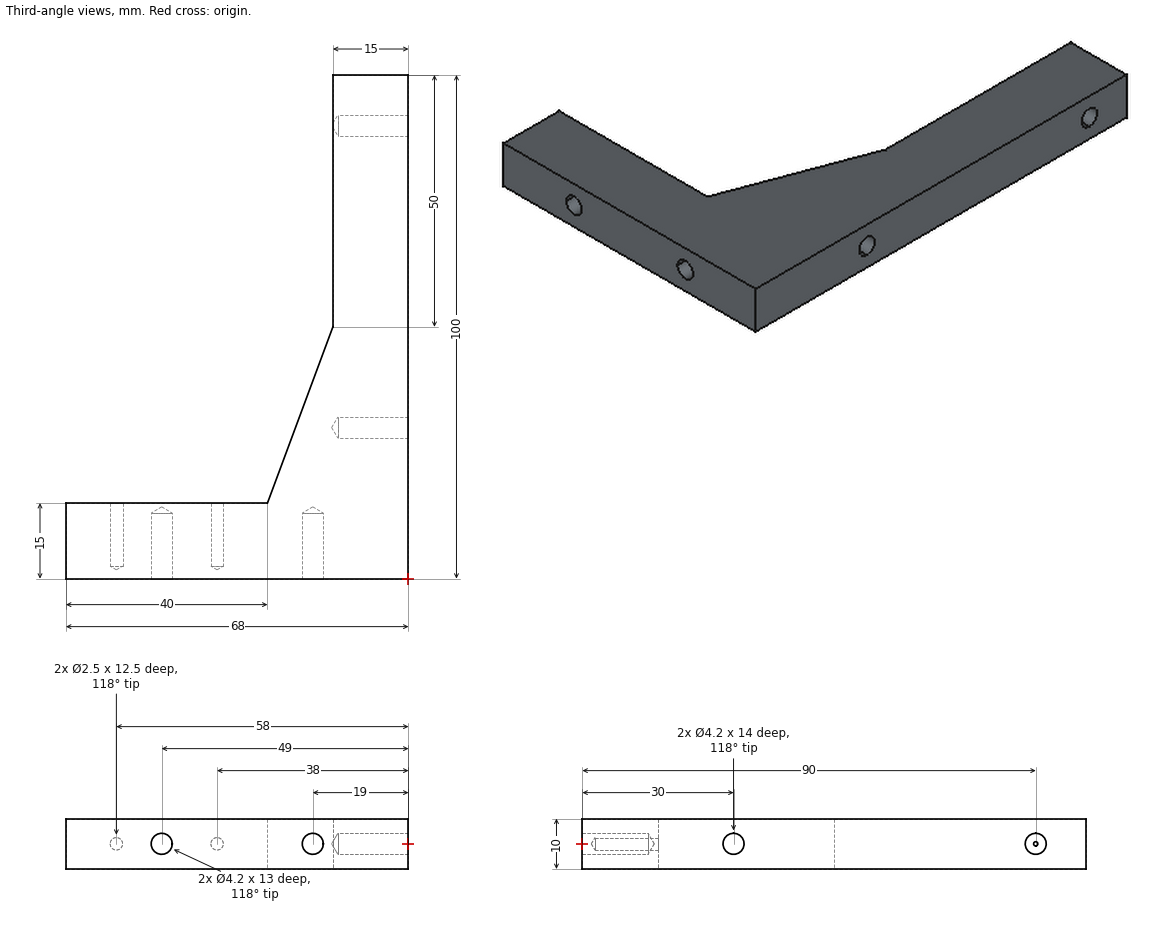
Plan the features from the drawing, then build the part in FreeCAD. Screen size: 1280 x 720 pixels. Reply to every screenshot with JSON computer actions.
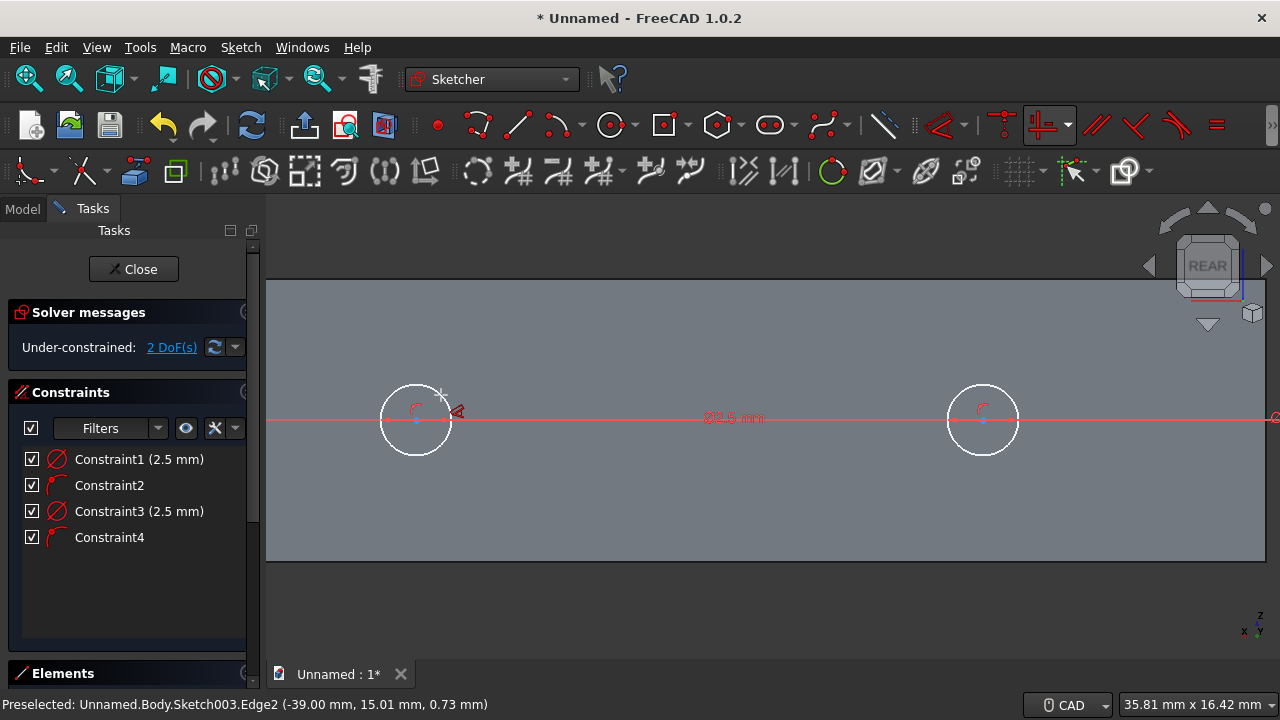
{"action": "left_click", "coordinate": [983, 420]}
{"action": "left_click", "coordinate": [638, 454]}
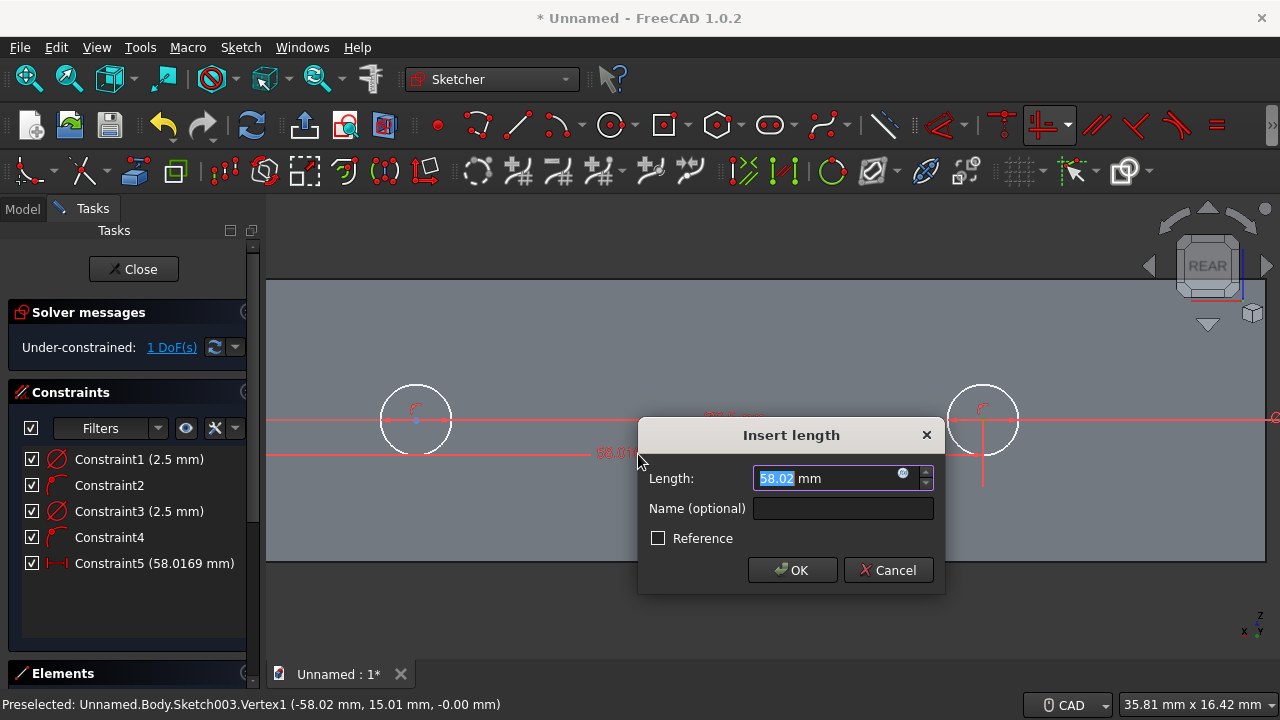
{"action": "type", "text": "58"}
{"action": "key", "text": "Return"}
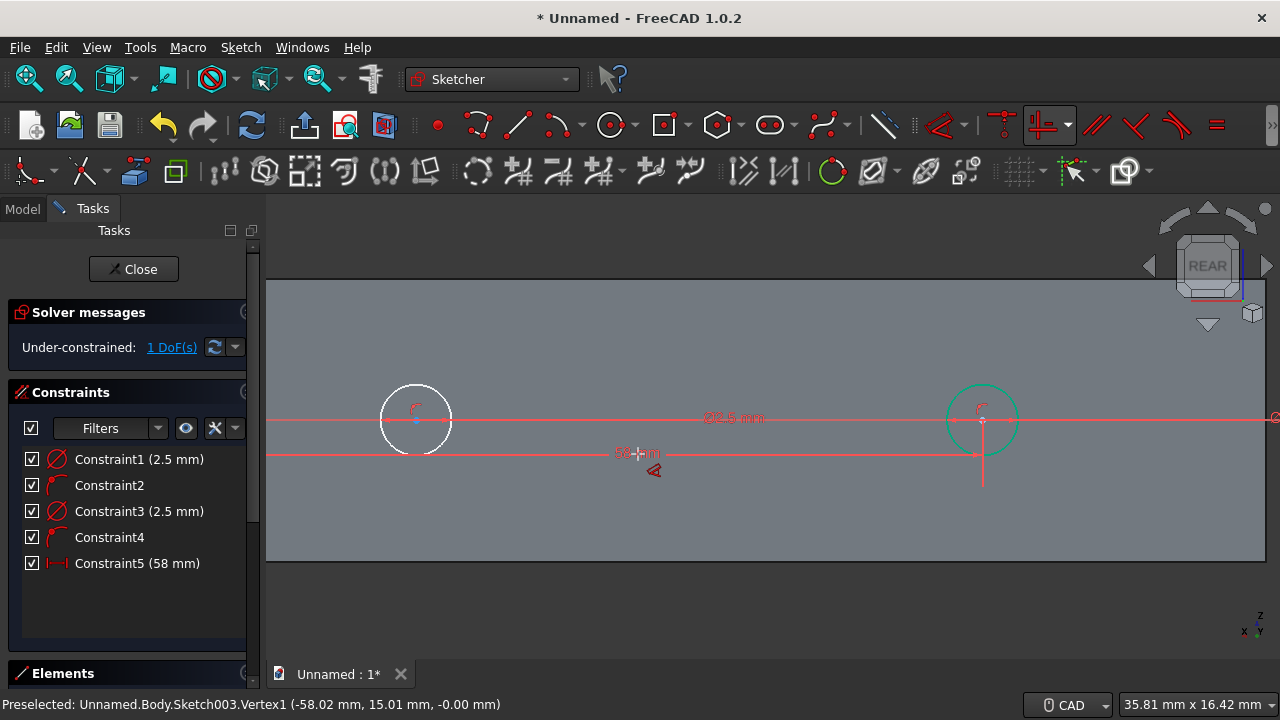
{"action": "left_click", "coordinate": [416, 420]}
{"action": "left_click", "coordinate": [355, 454]}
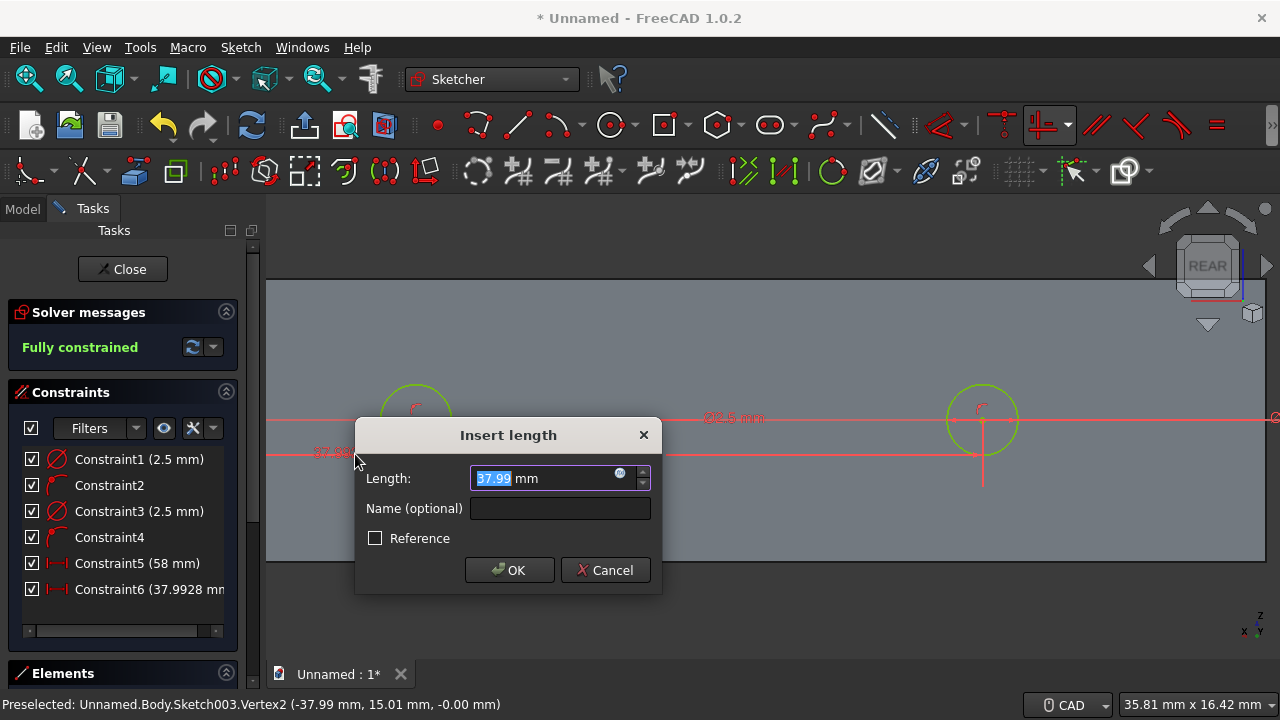
{"action": "type", "text": "38"}
{"action": "key", "text": "Return"}
{"action": "key", "text": "Escape"}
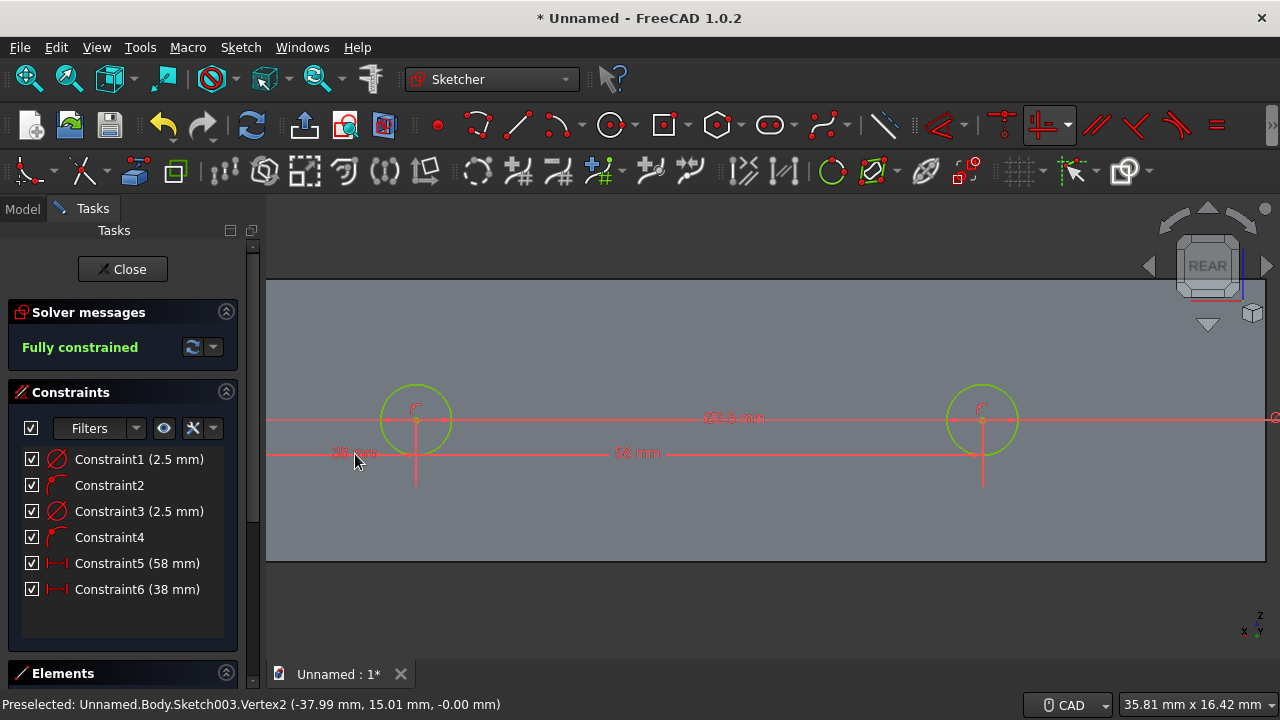
{"action": "left_click", "coordinate": [123, 269]}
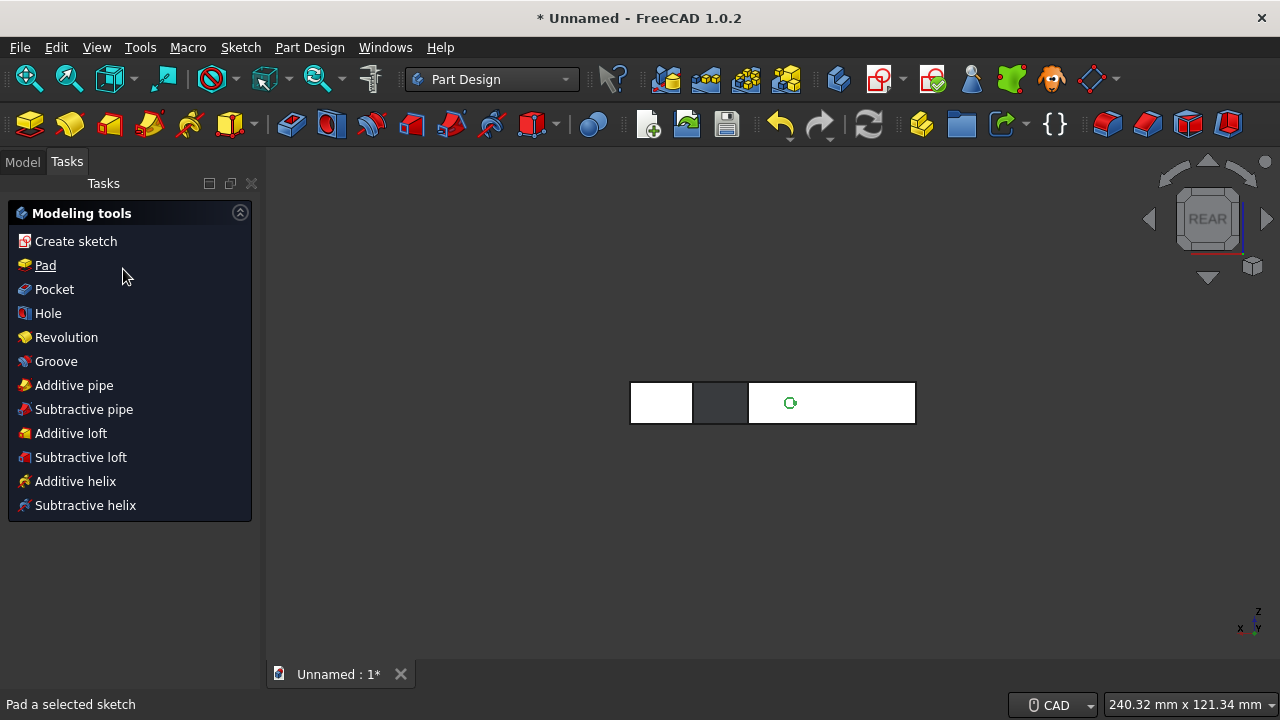
{"action": "left_click", "coordinate": [332, 124]}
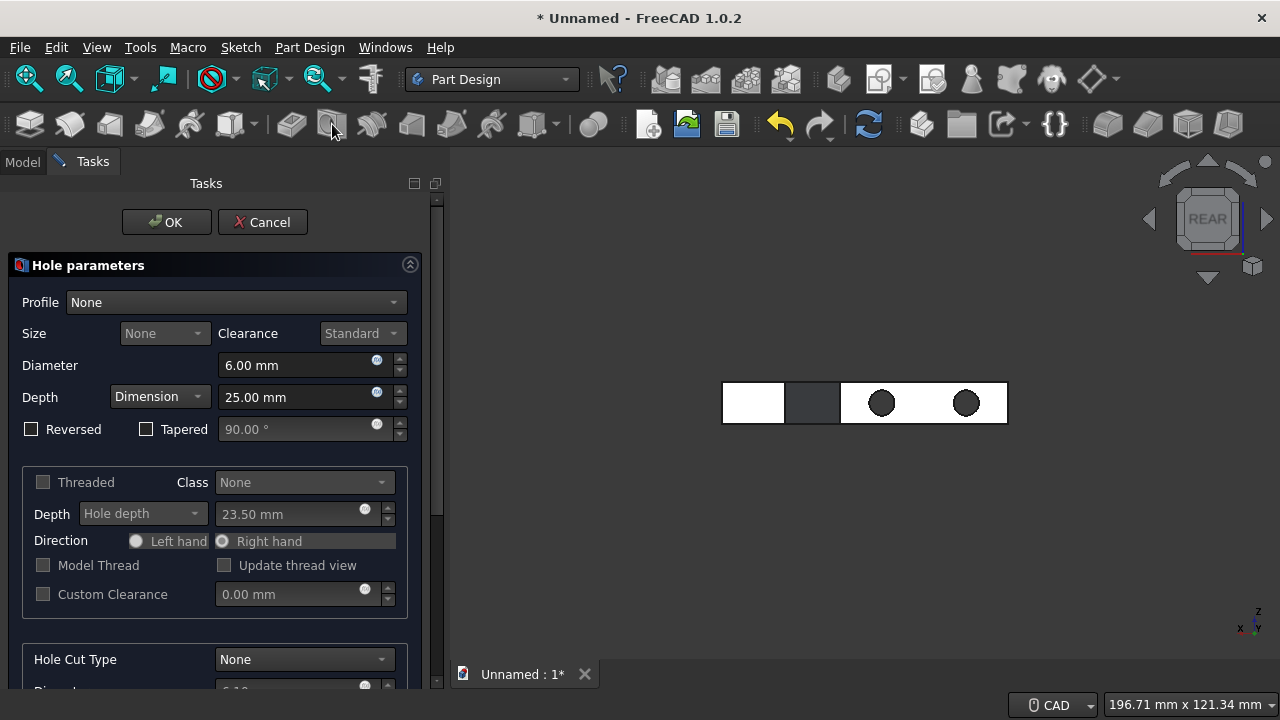
{"action": "triple_click", "coordinate": [305, 365]}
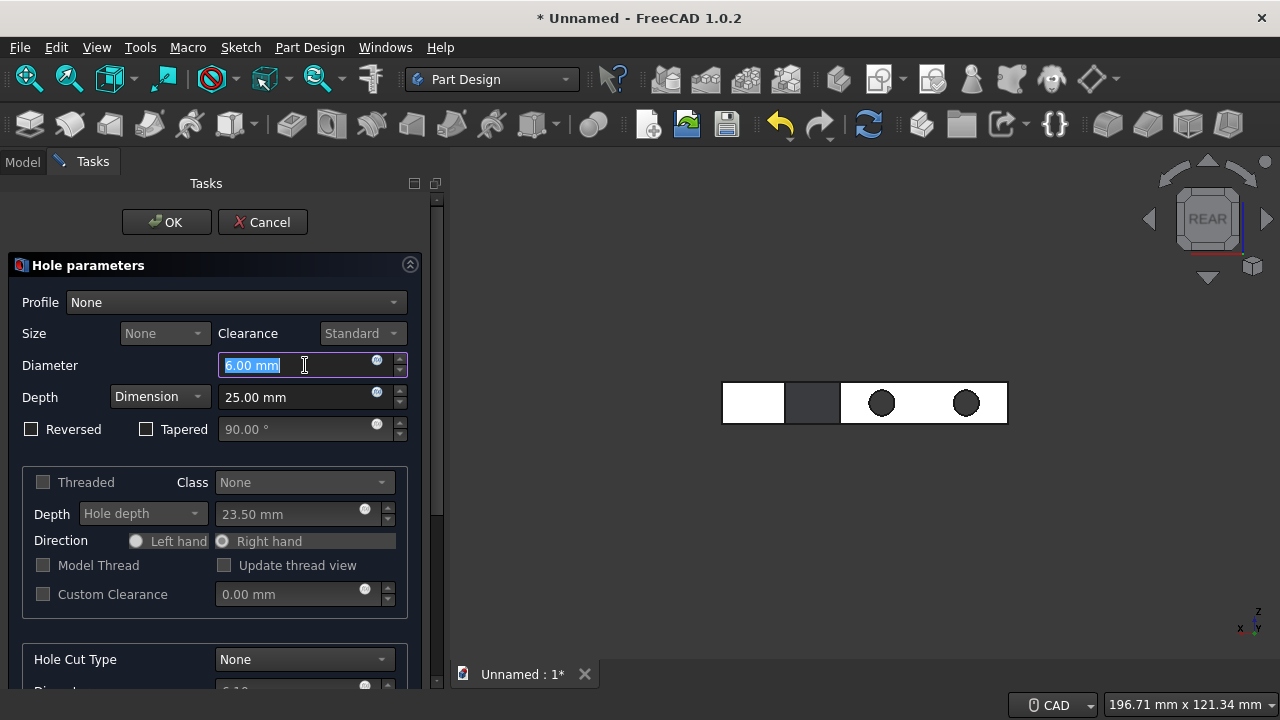
{"action": "type", "text": "2.5"}
{"action": "key", "text": "Tab"}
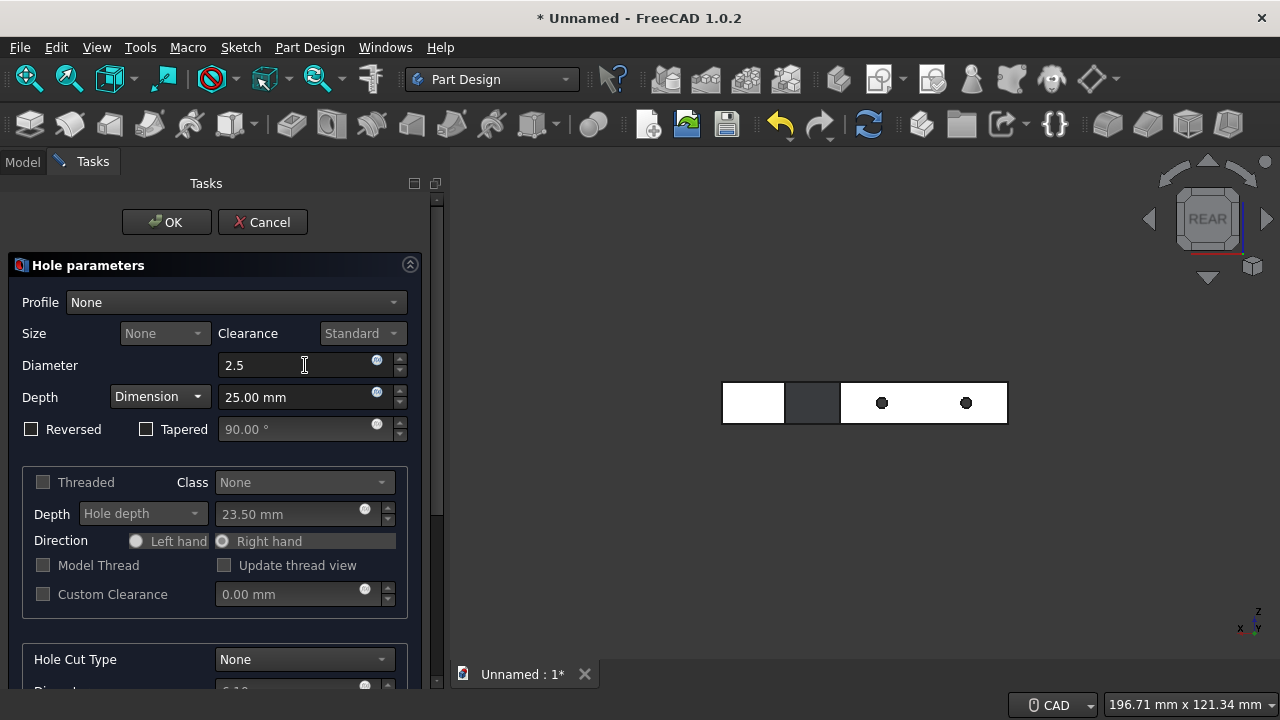
{"action": "triple_click", "coordinate": [305, 397]}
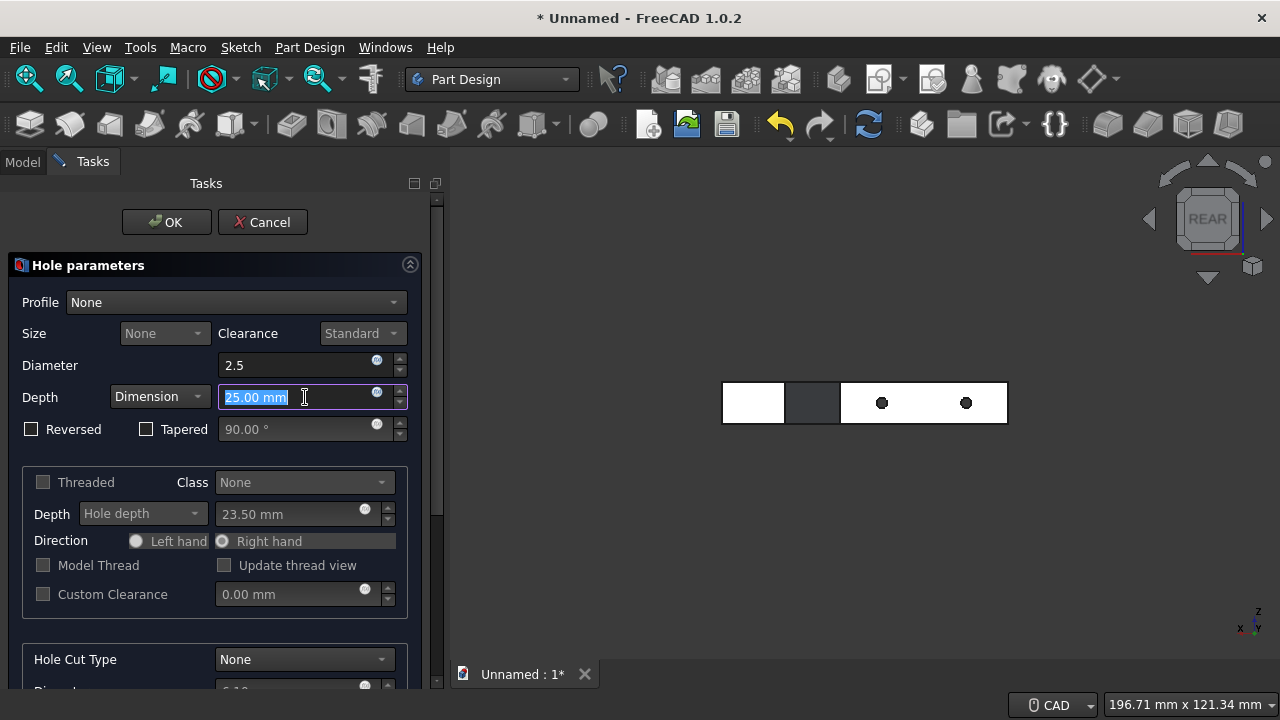
{"action": "type", "text": "12.5"}
{"action": "key", "text": "Tab"}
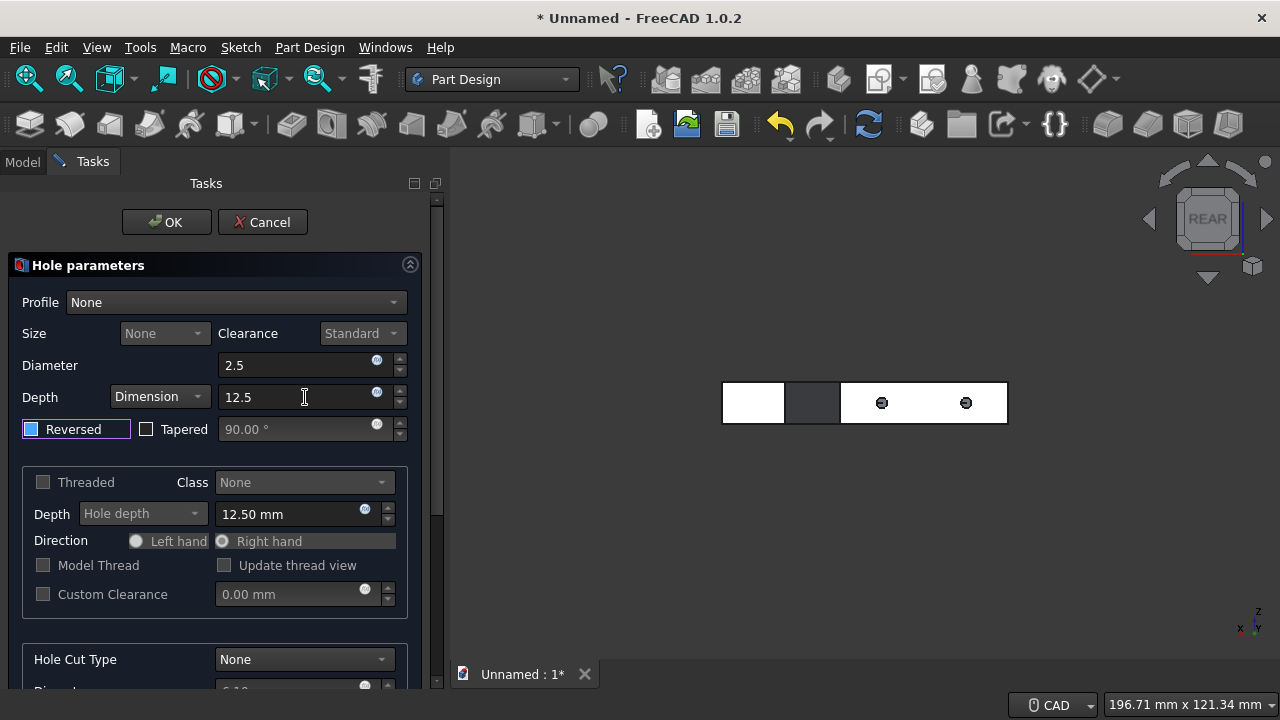
{"action": "left_click", "coordinate": [167, 222]}